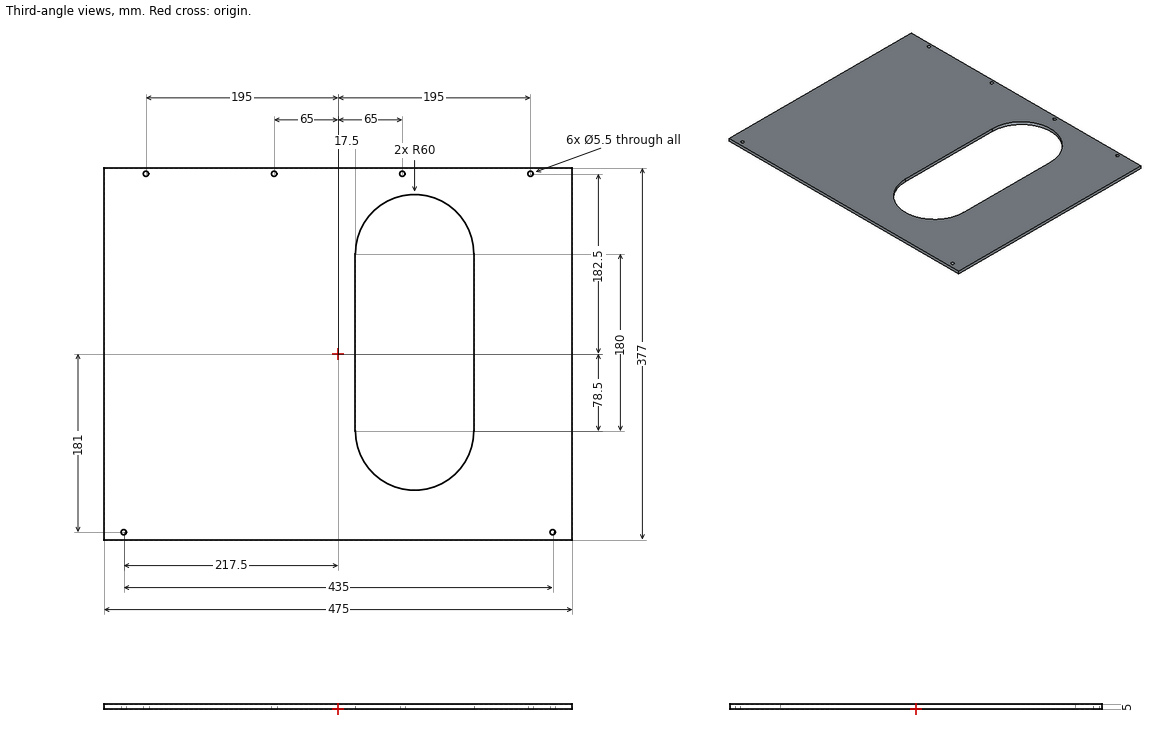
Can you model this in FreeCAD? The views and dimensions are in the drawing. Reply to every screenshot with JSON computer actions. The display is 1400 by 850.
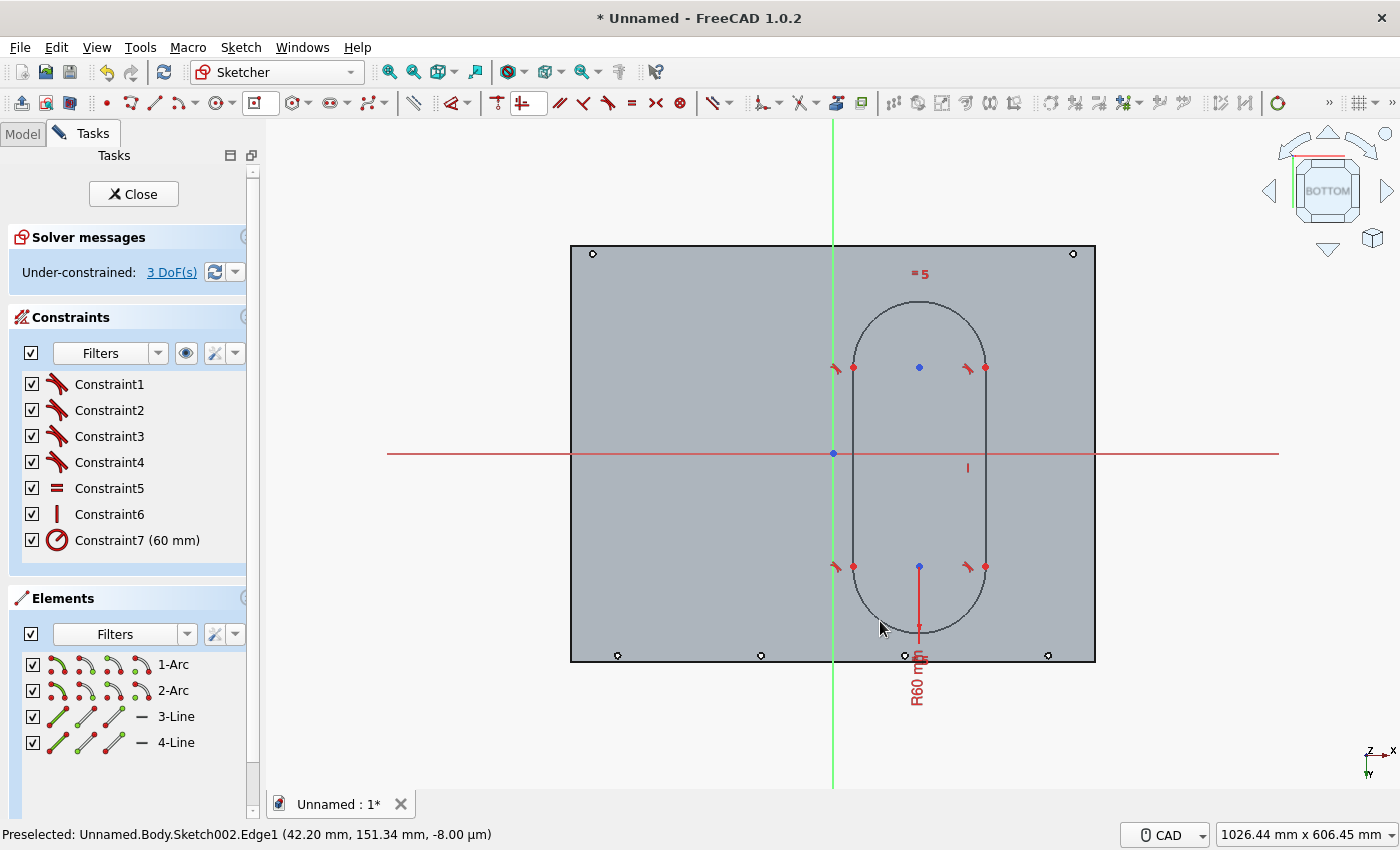
{"action": "left_click", "coordinate": [853, 507]}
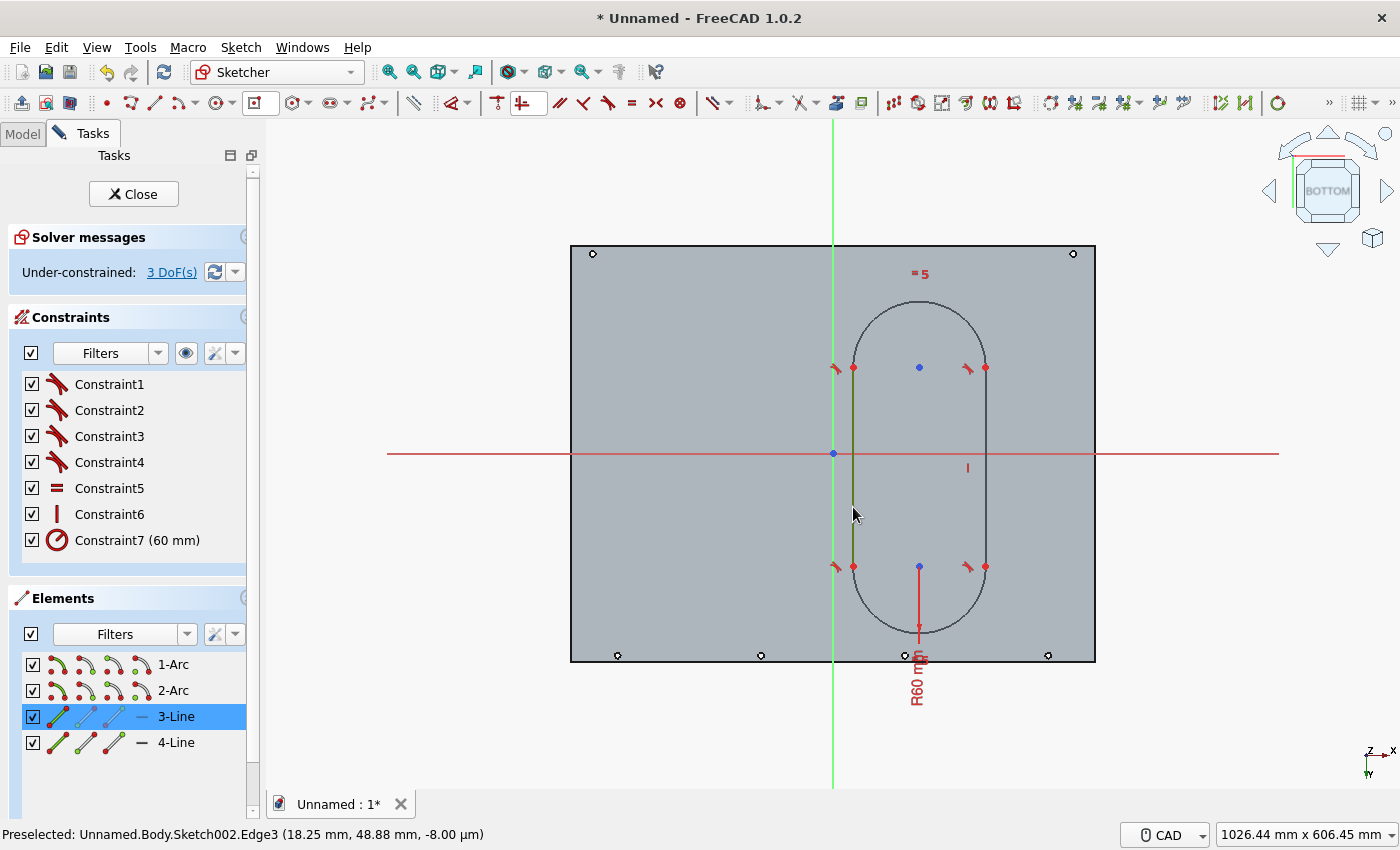
{"action": "key", "text": "i"}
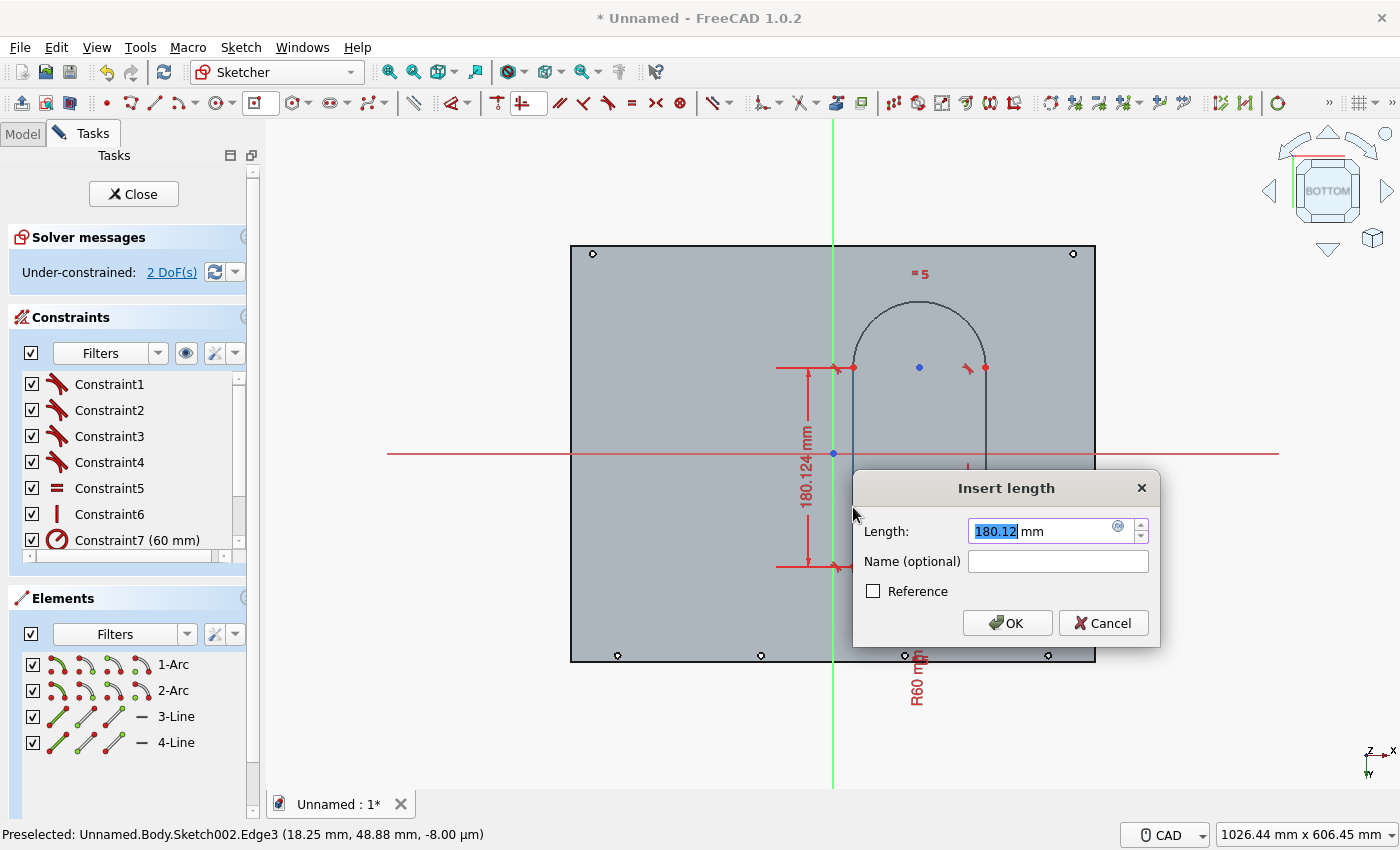
{"action": "type", "text": "180"}
{"action": "key", "text": "Return"}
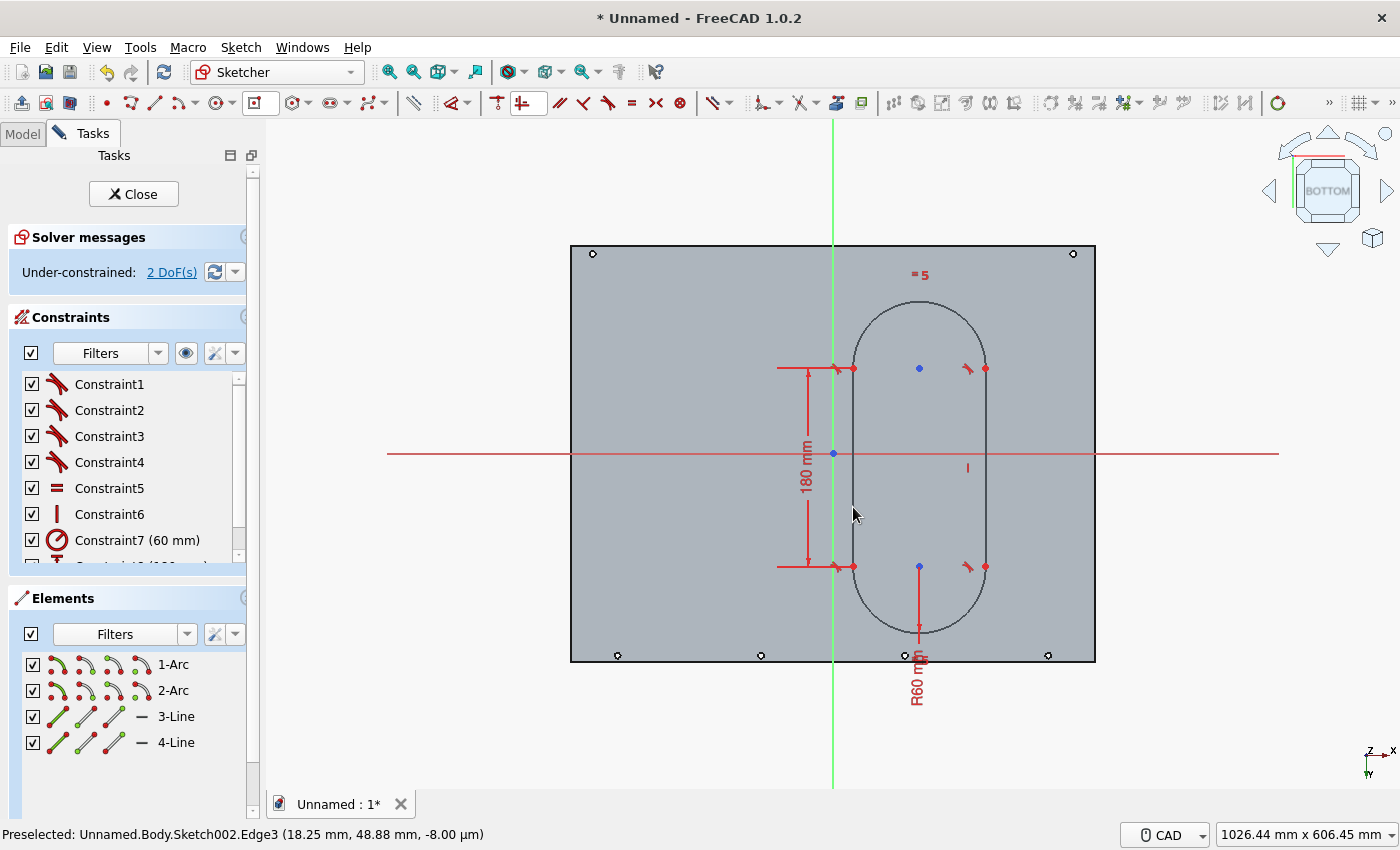
{"action": "scroll", "coordinate": [853, 567], "scroll_direction": "up", "scroll_amount": 4}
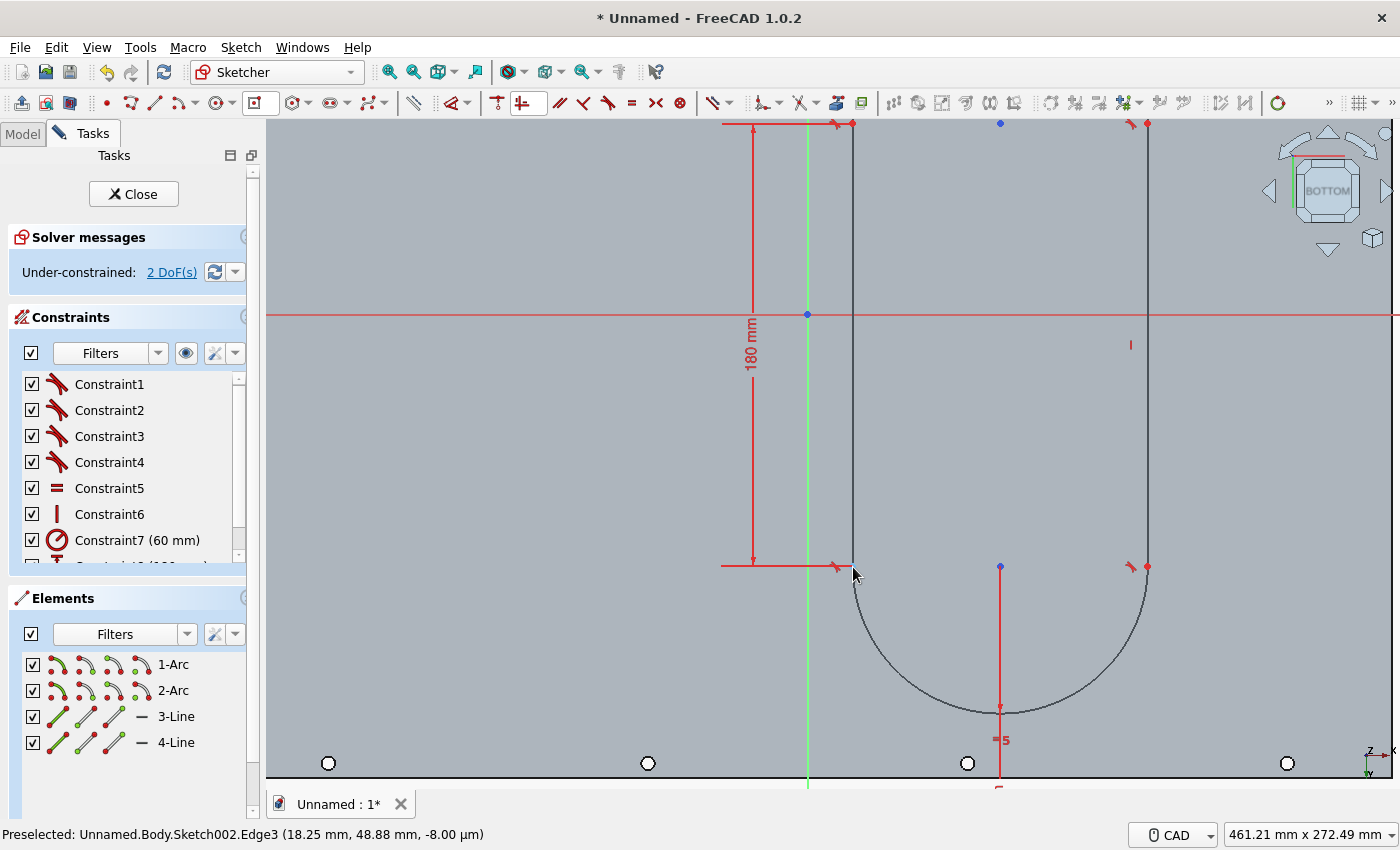
{"action": "left_click", "coordinate": [853, 566]}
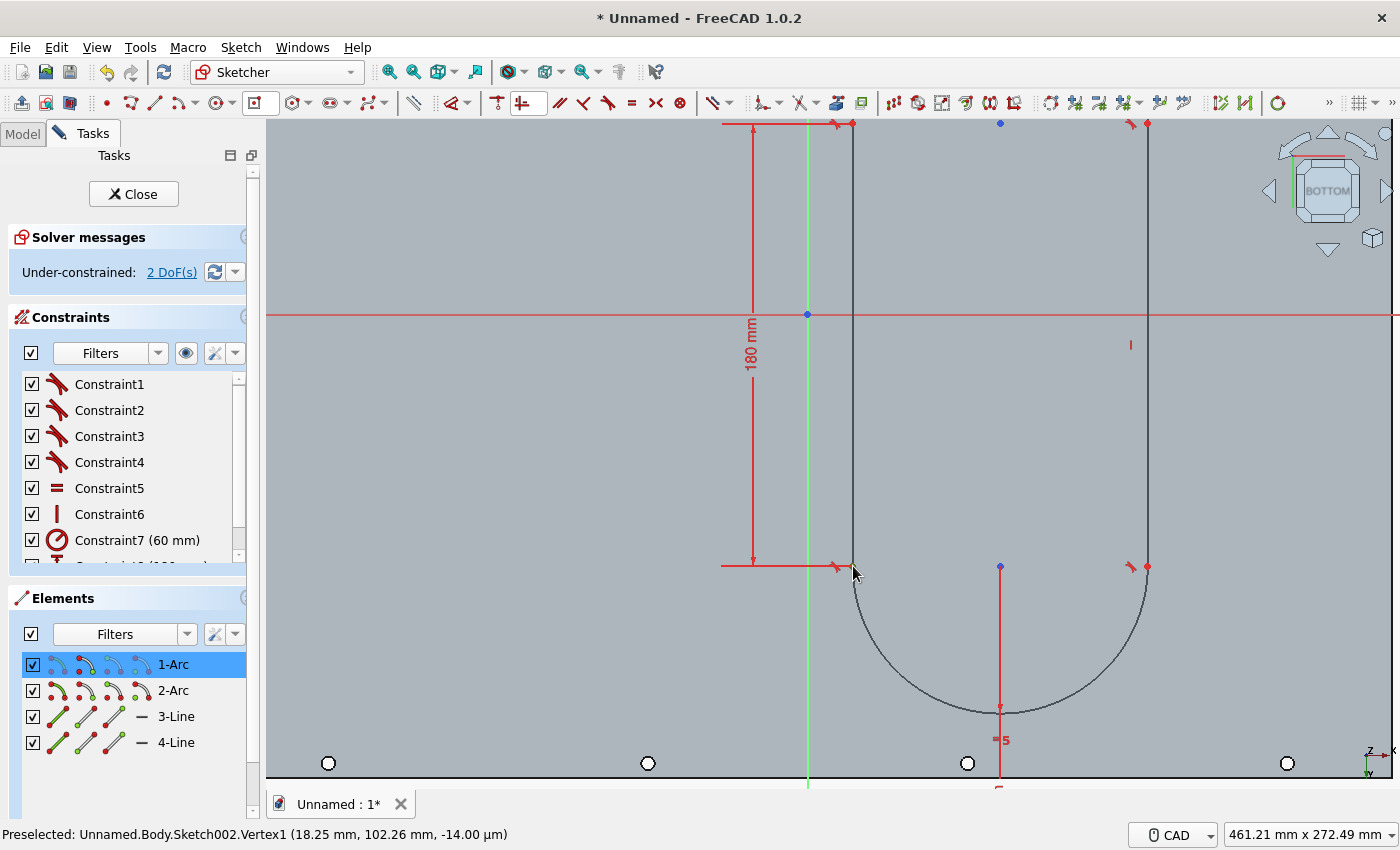
{"action": "left_click", "coordinate": [470, 104]}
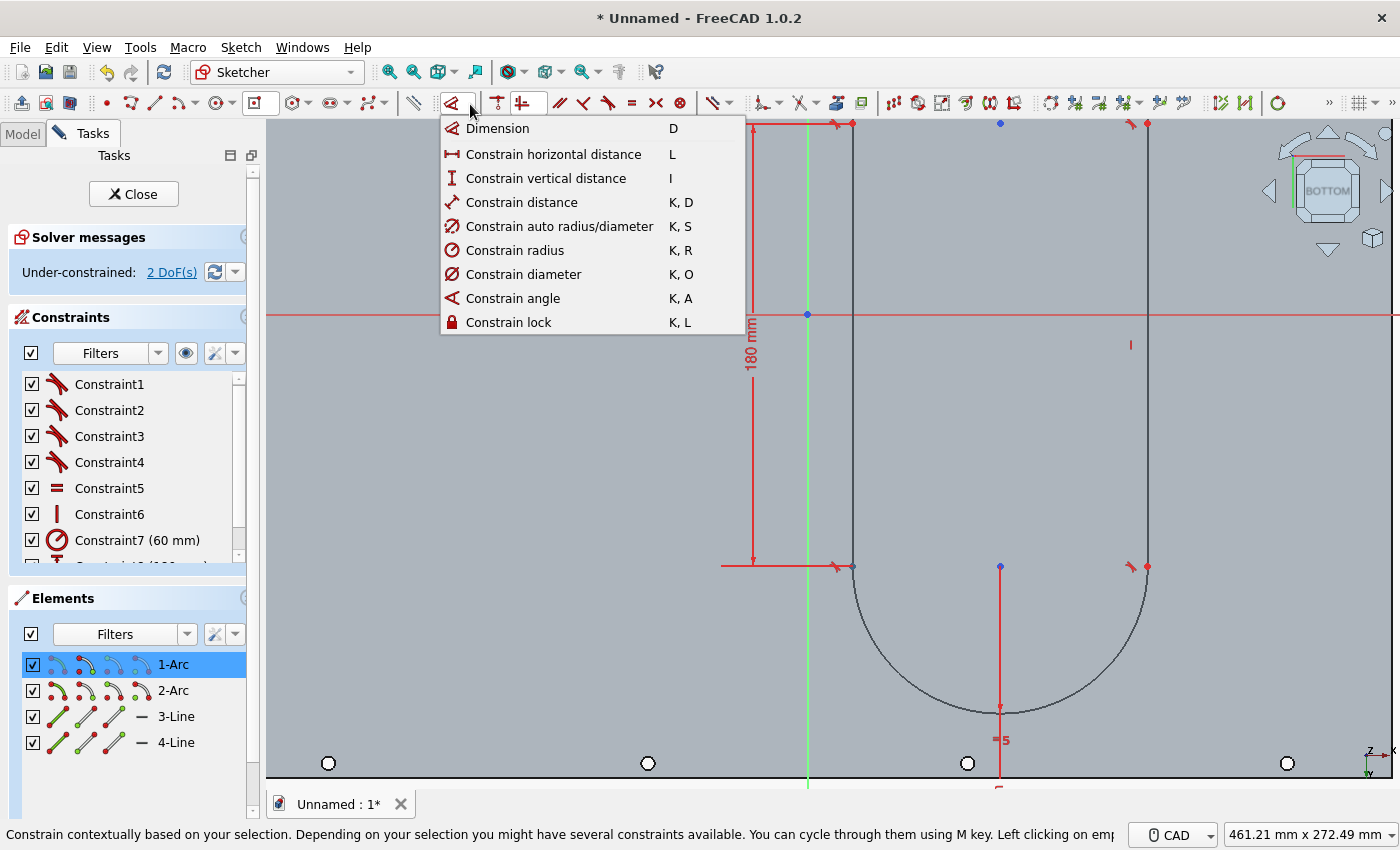
{"action": "left_click", "coordinate": [593, 154]}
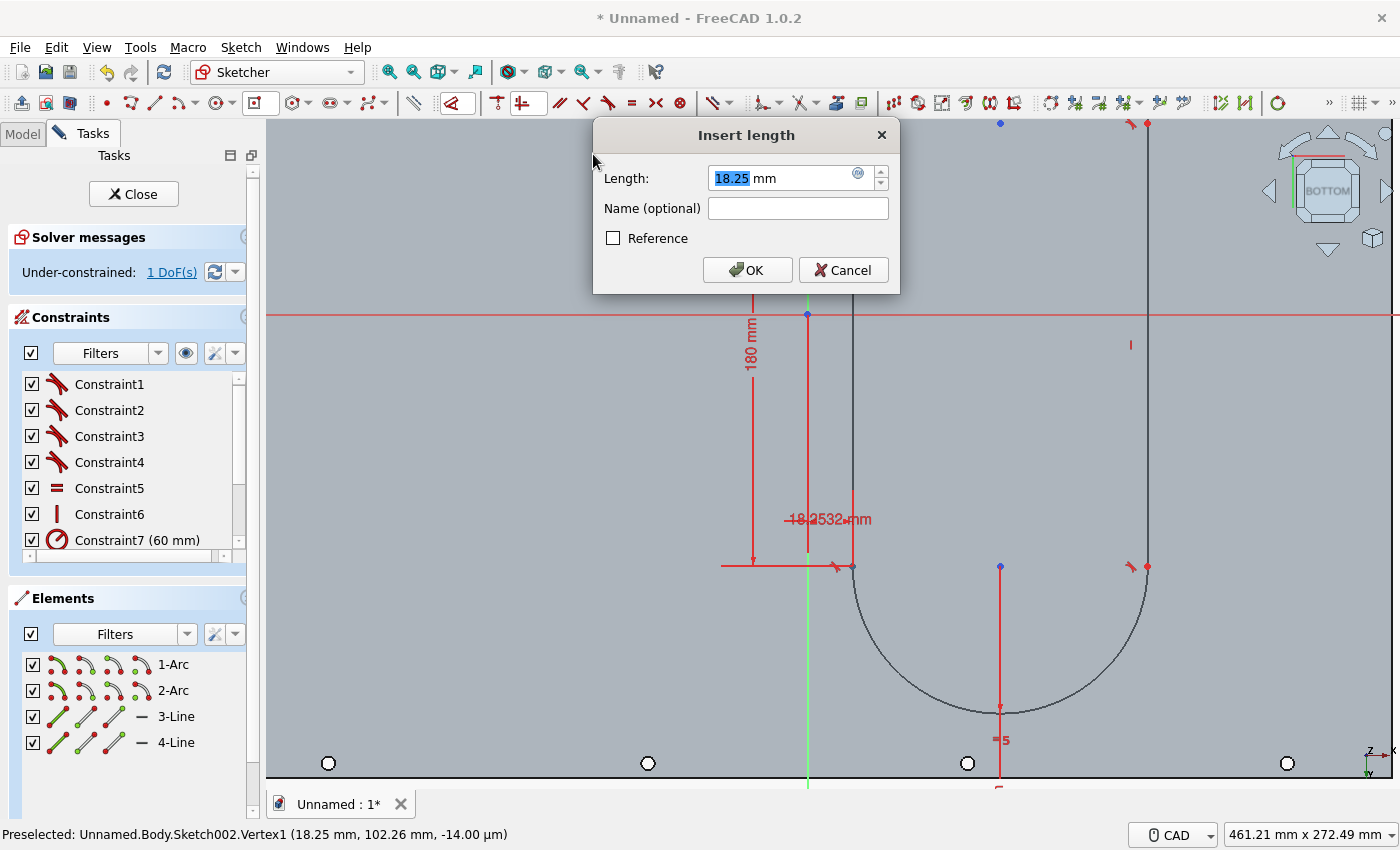
{"action": "type", "text": "17.5"}
{"action": "key", "text": "Return"}